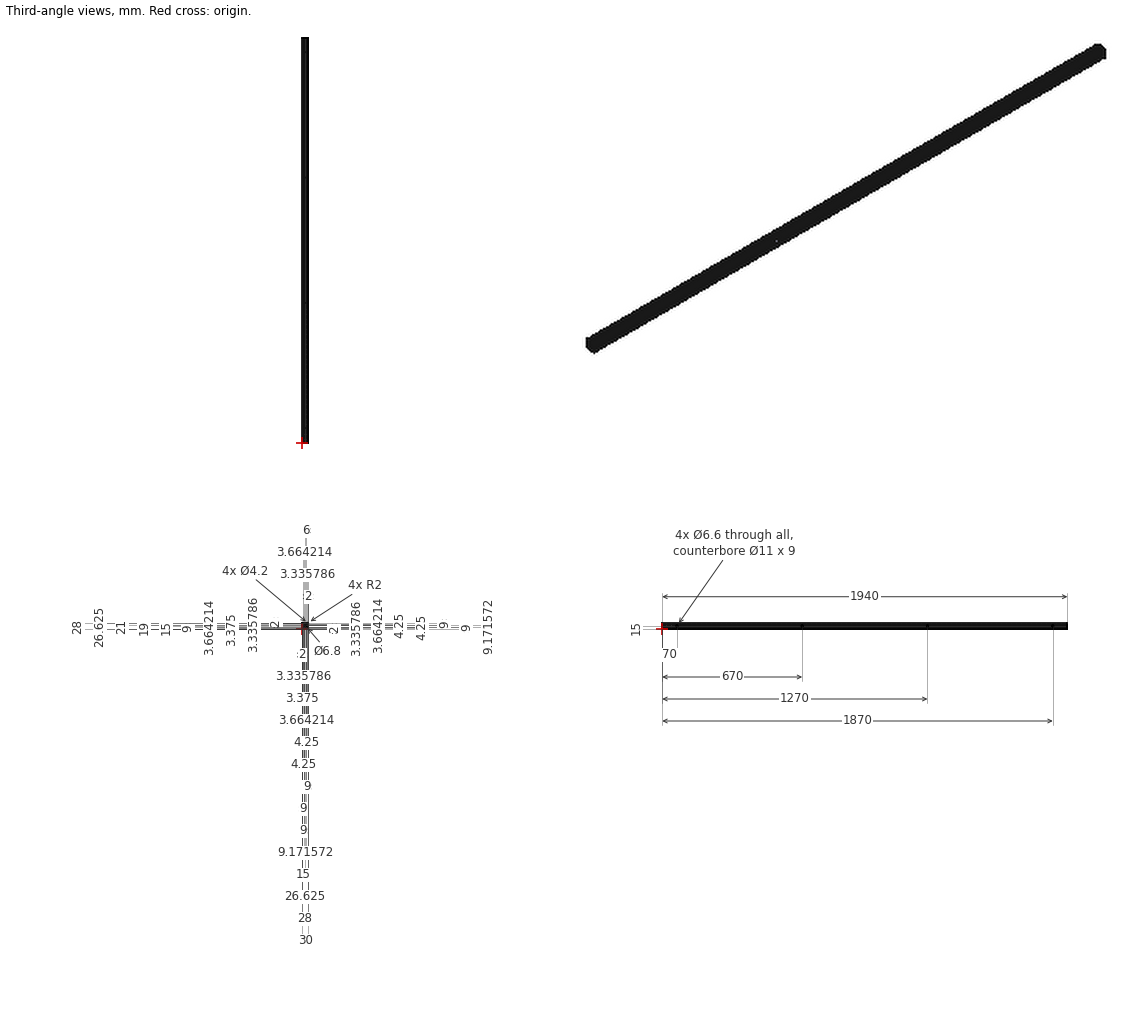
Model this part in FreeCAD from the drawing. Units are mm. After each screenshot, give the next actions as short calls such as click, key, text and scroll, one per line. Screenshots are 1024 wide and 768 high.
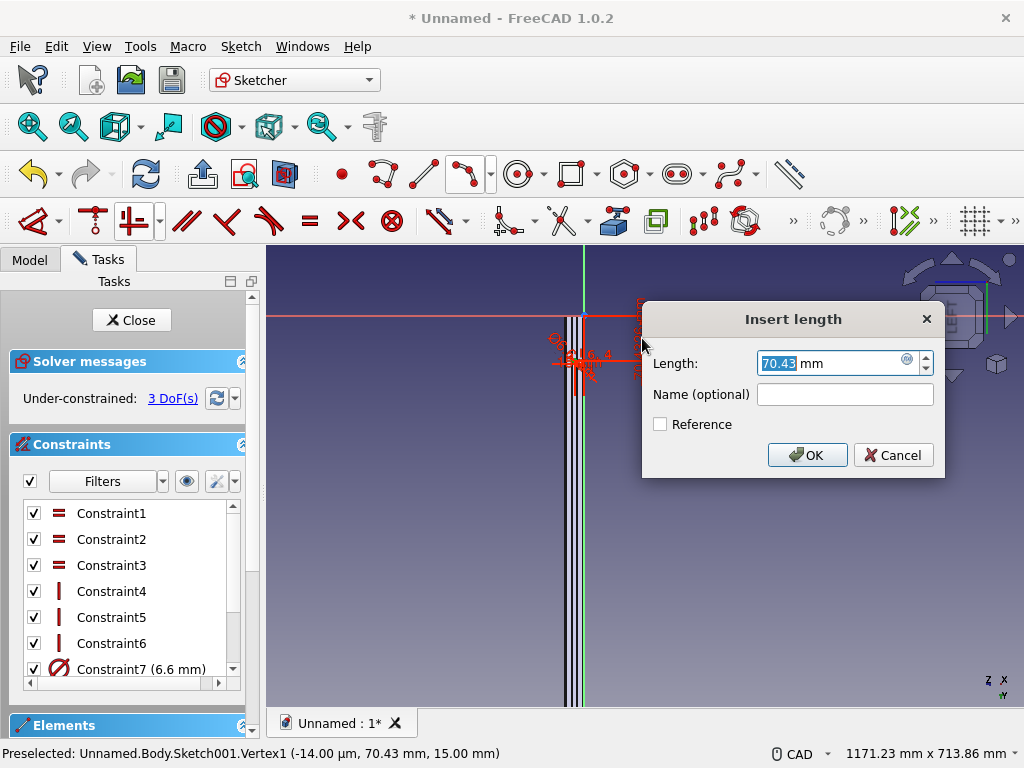
text(70)
key(Return)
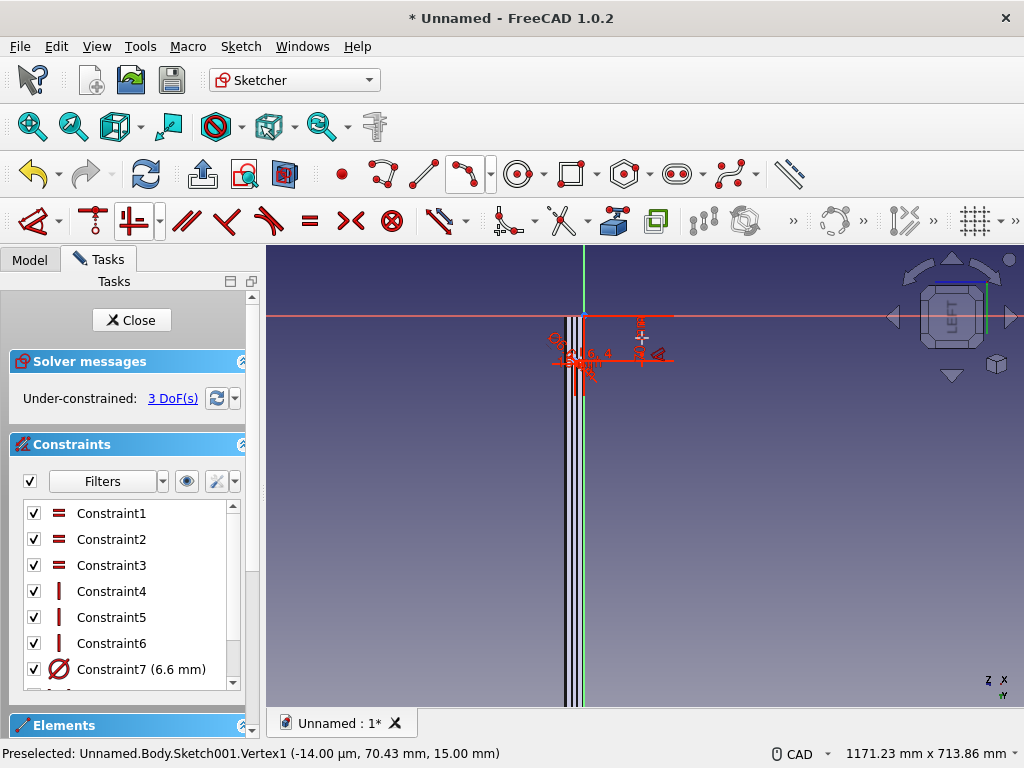
scroll(576, 330, down, 7)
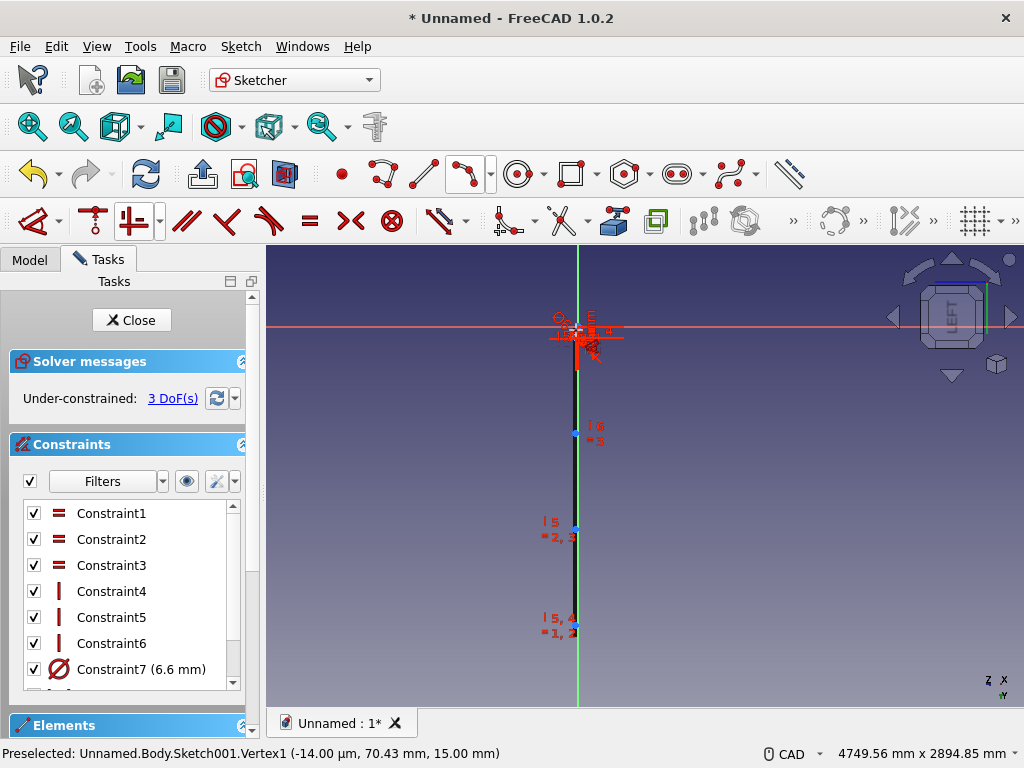
click(576, 434)
click(612, 380)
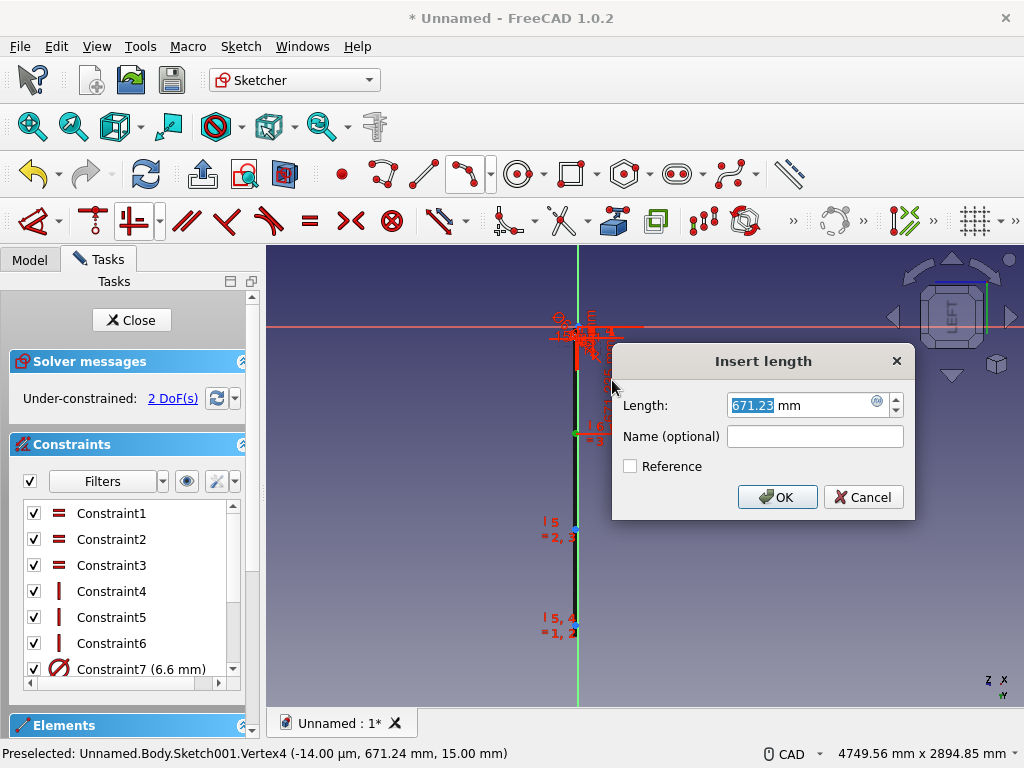
text(670)
key(Return)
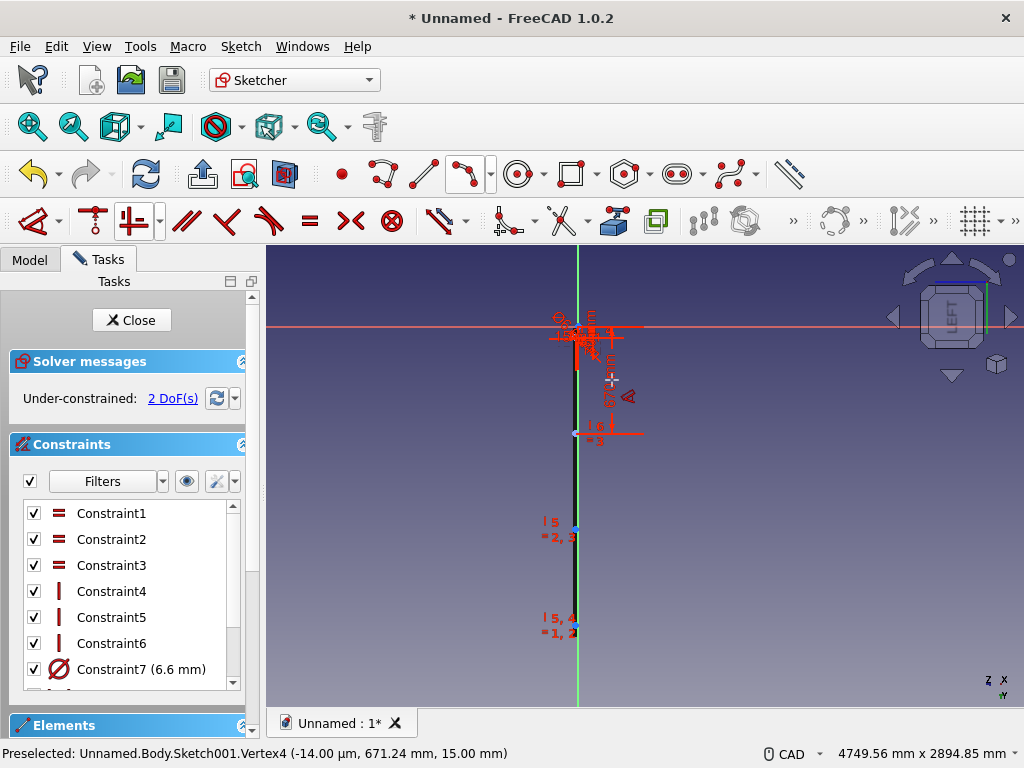
click(576, 625)
click(612, 476)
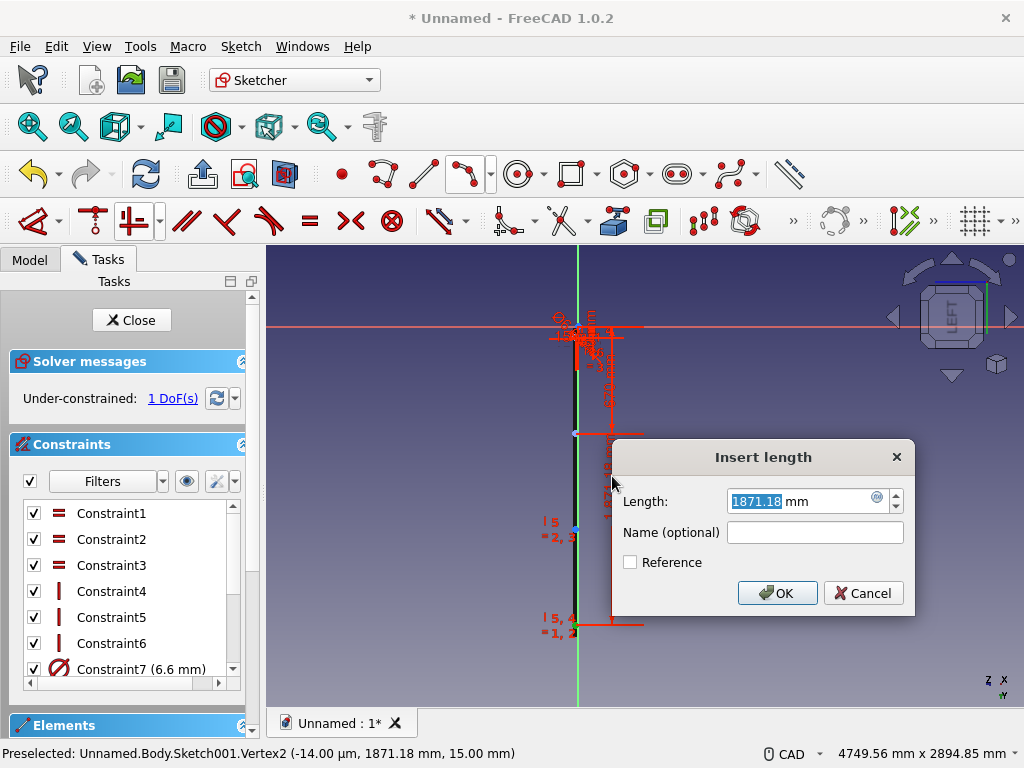
text(1870)
key(Return)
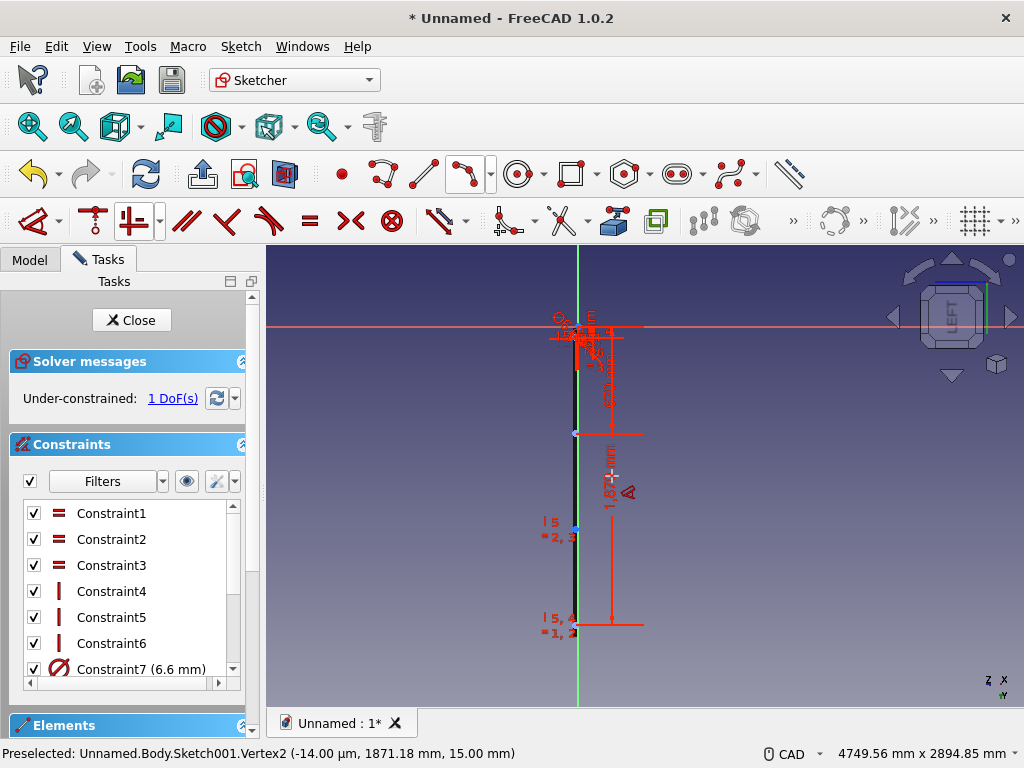
click(576, 529)
click(612, 428)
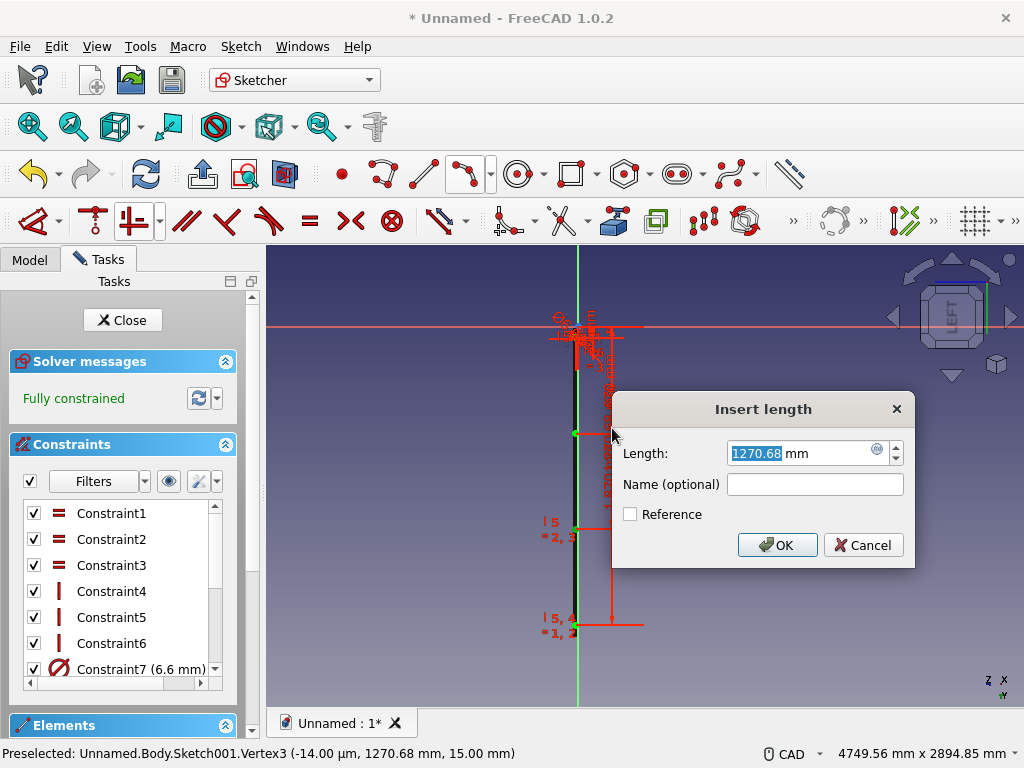
text(1270)
key(Return)
key(Escape)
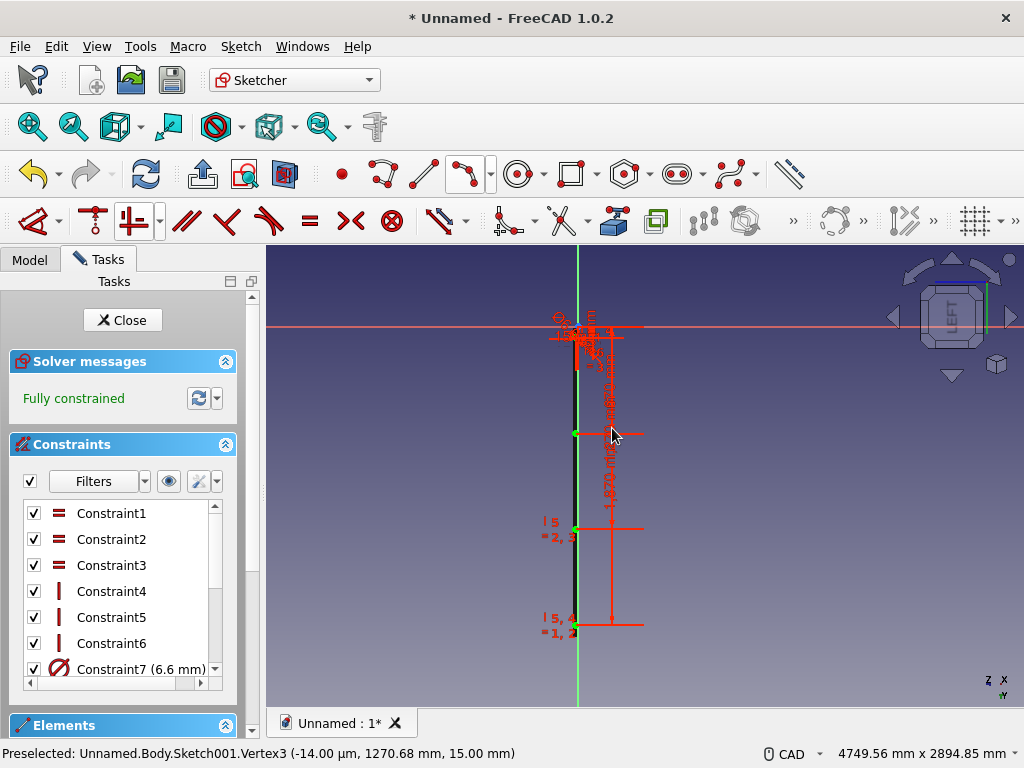
click(123, 320)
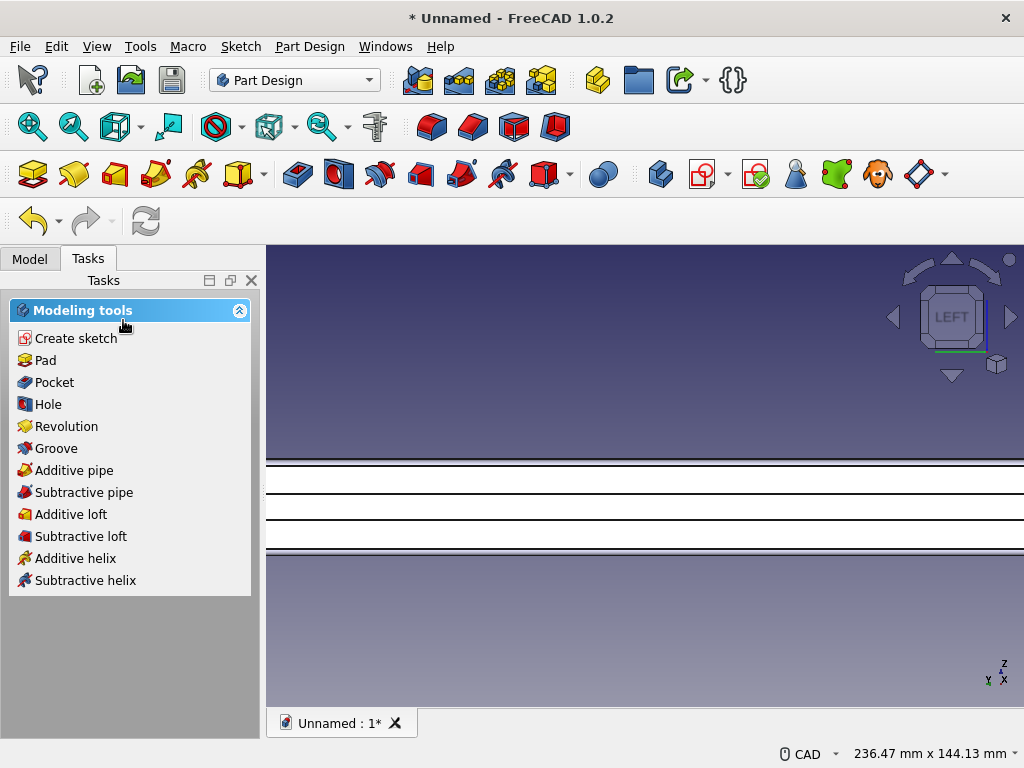
click(339, 174)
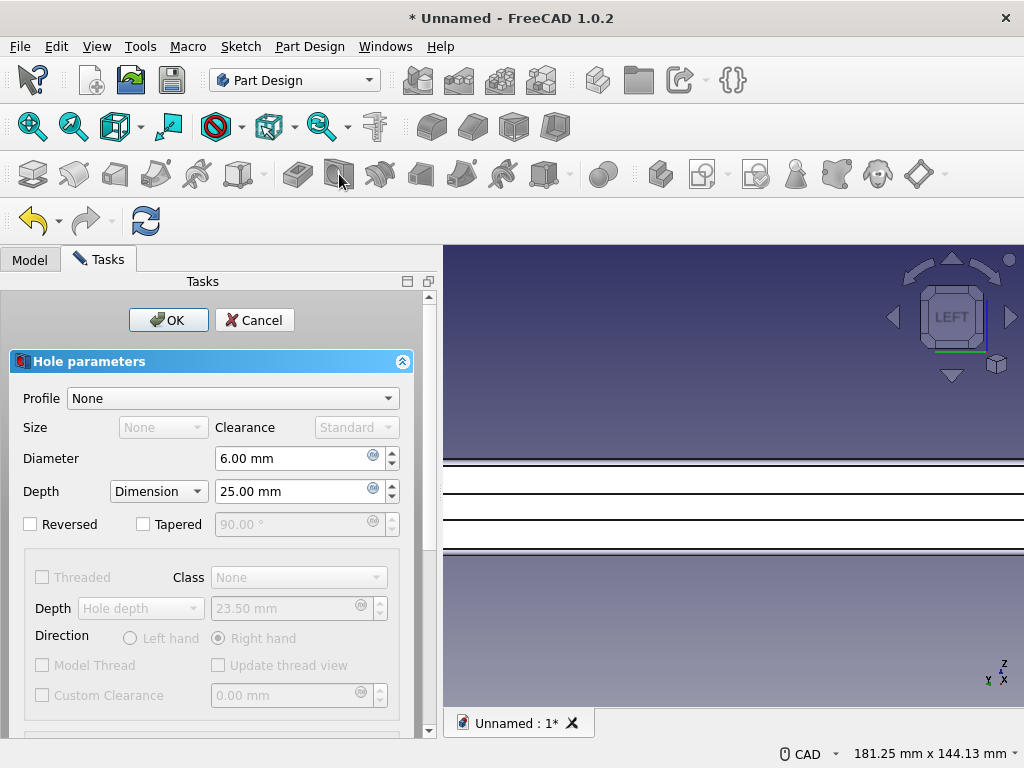
triple_click(300, 458)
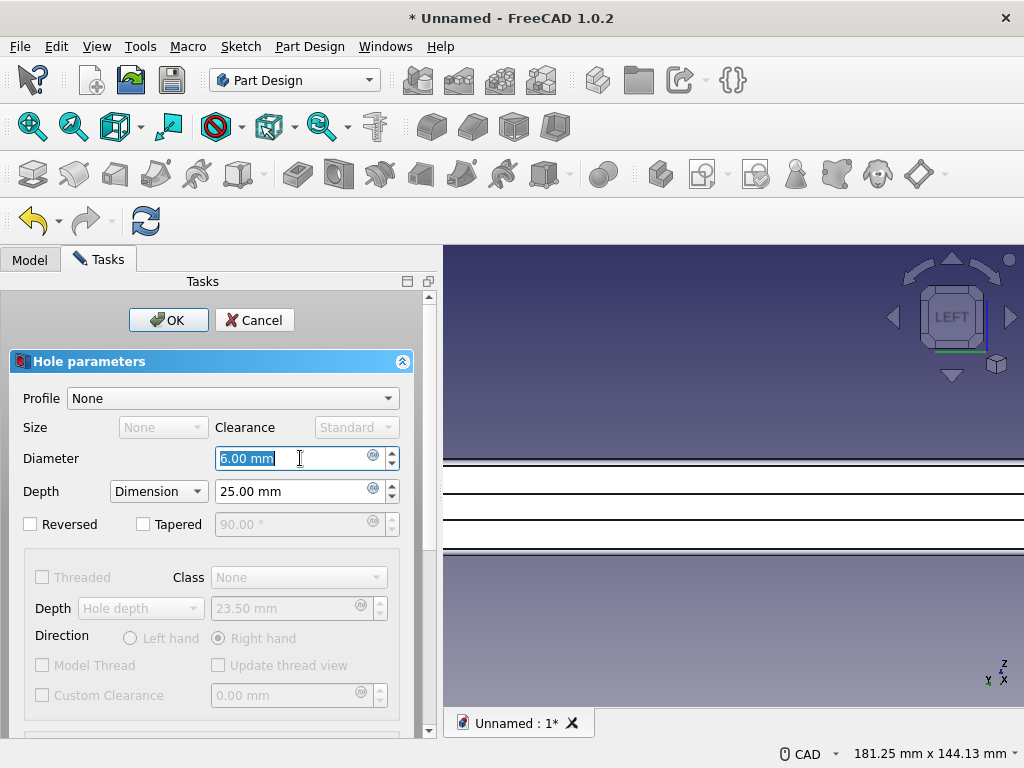
text(6.6)
key(Tab)